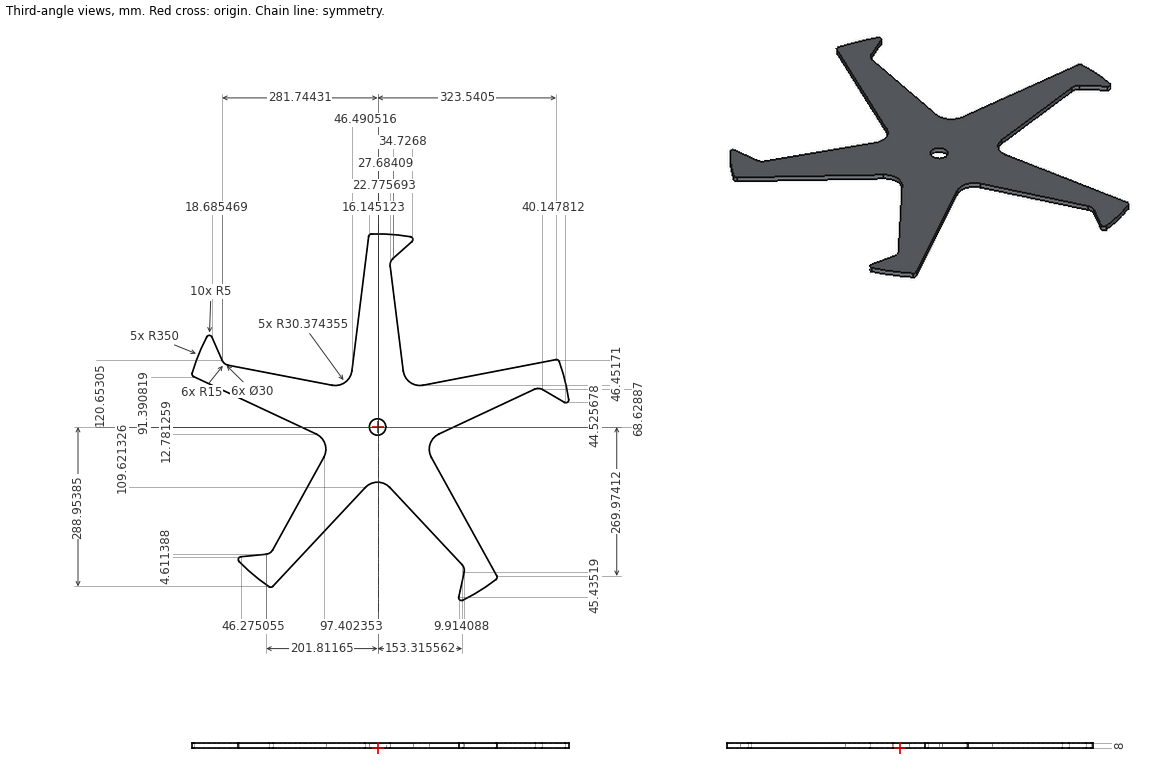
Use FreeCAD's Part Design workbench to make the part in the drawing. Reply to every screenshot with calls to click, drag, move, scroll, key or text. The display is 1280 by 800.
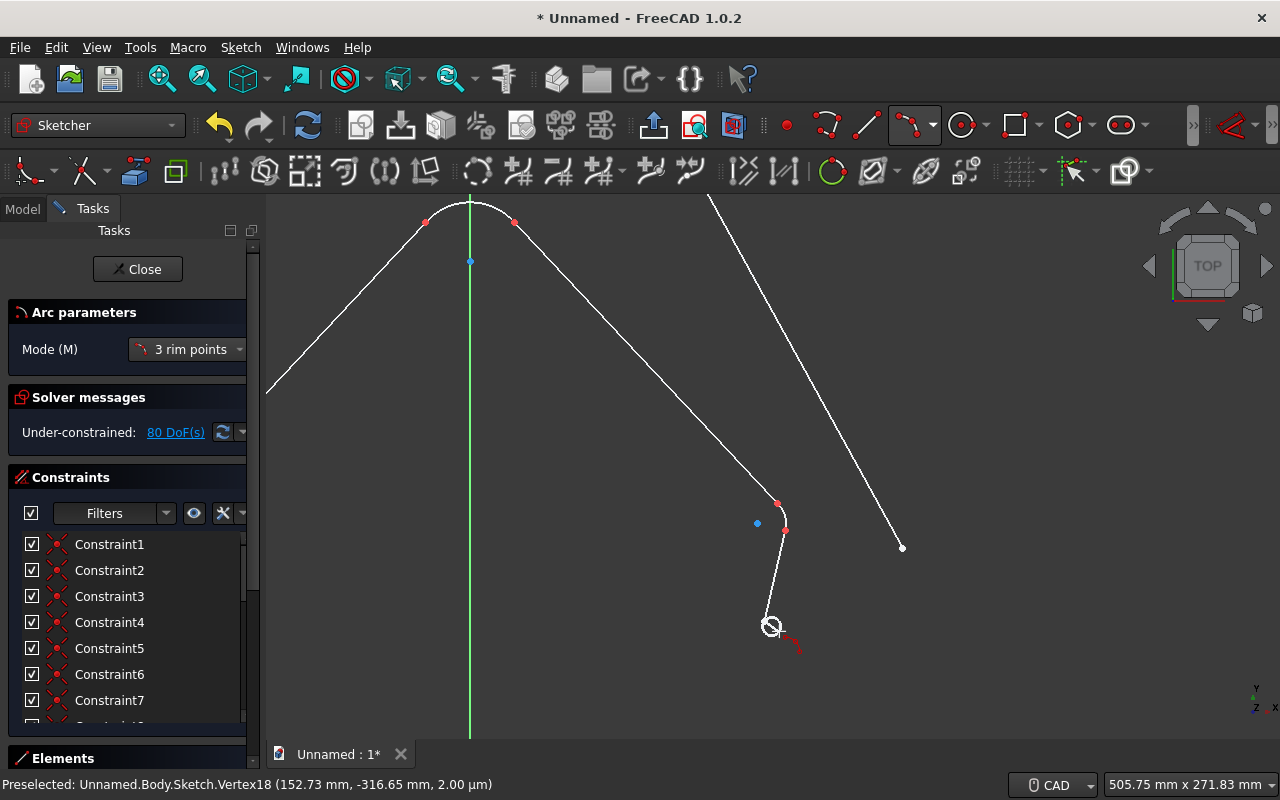
scroll(769, 630, up, 6)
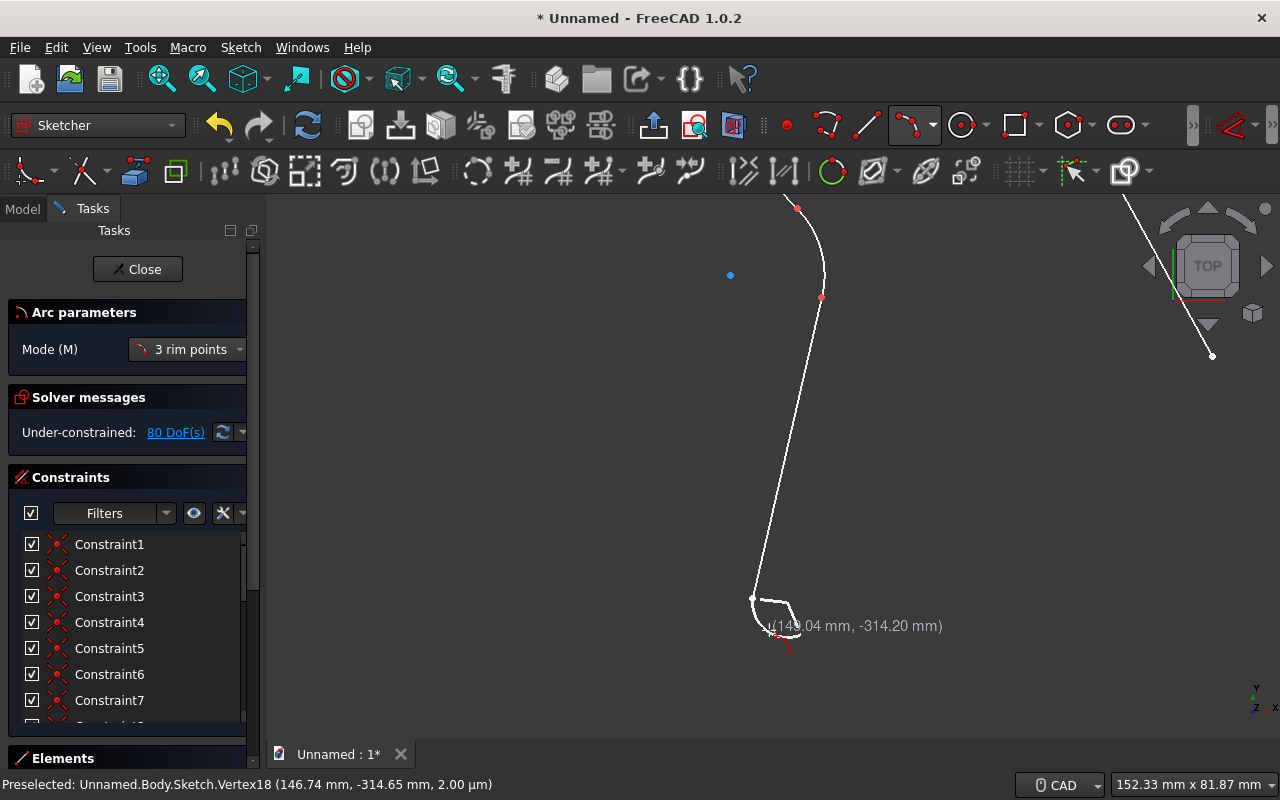
click(767, 628)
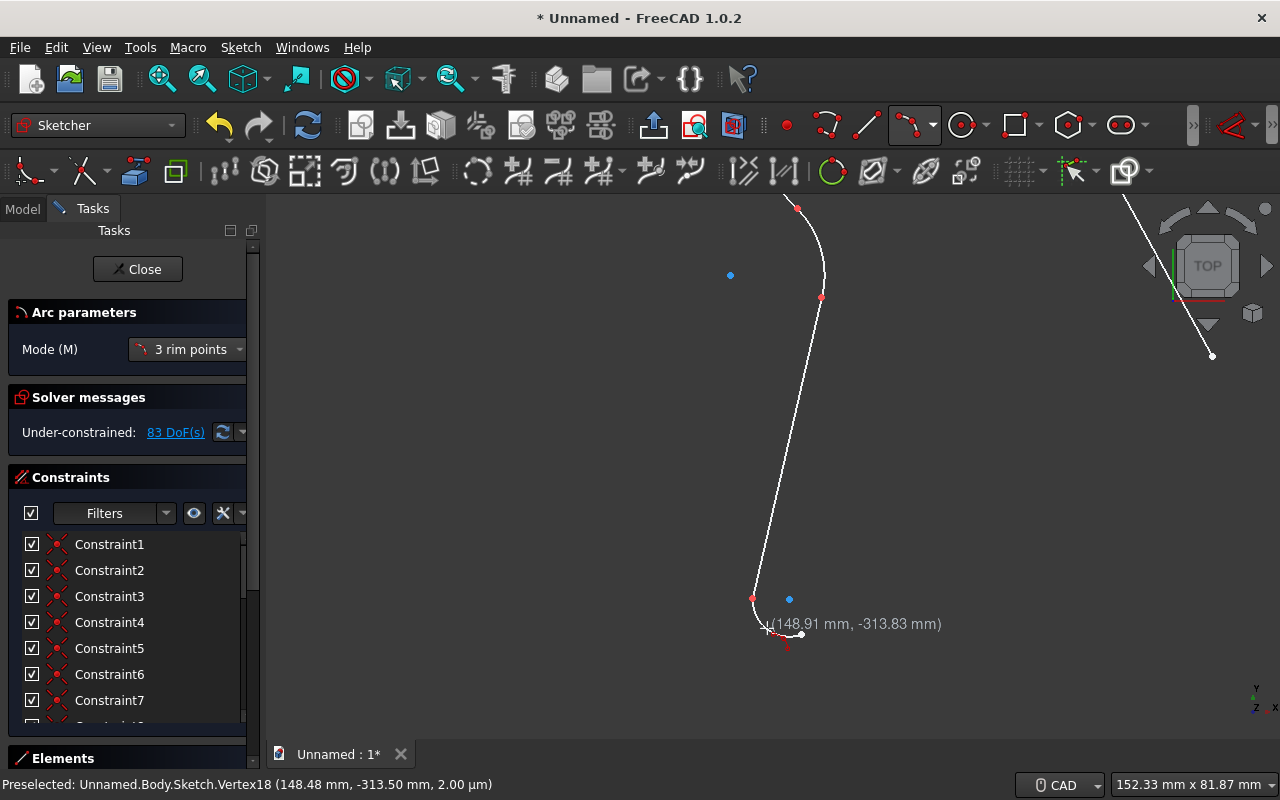
click(801, 635)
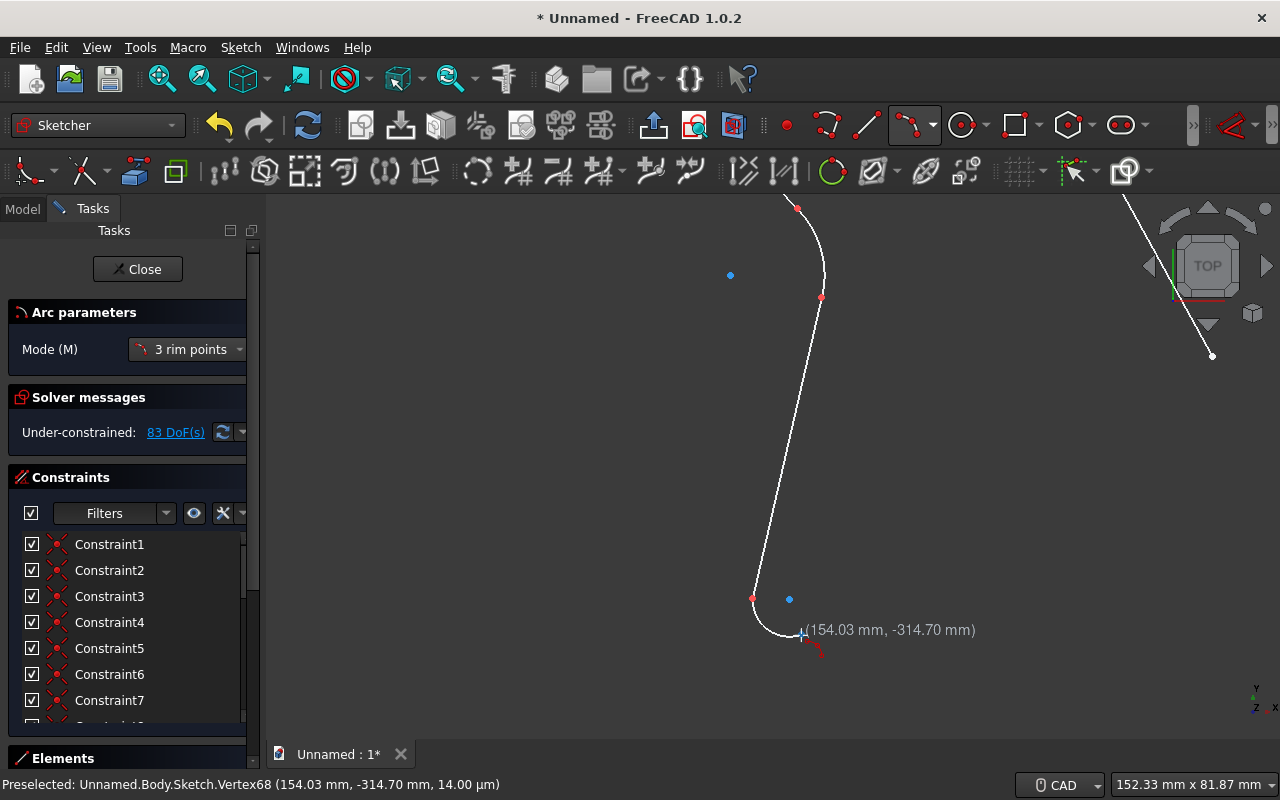
scroll(776, 631, down, 13)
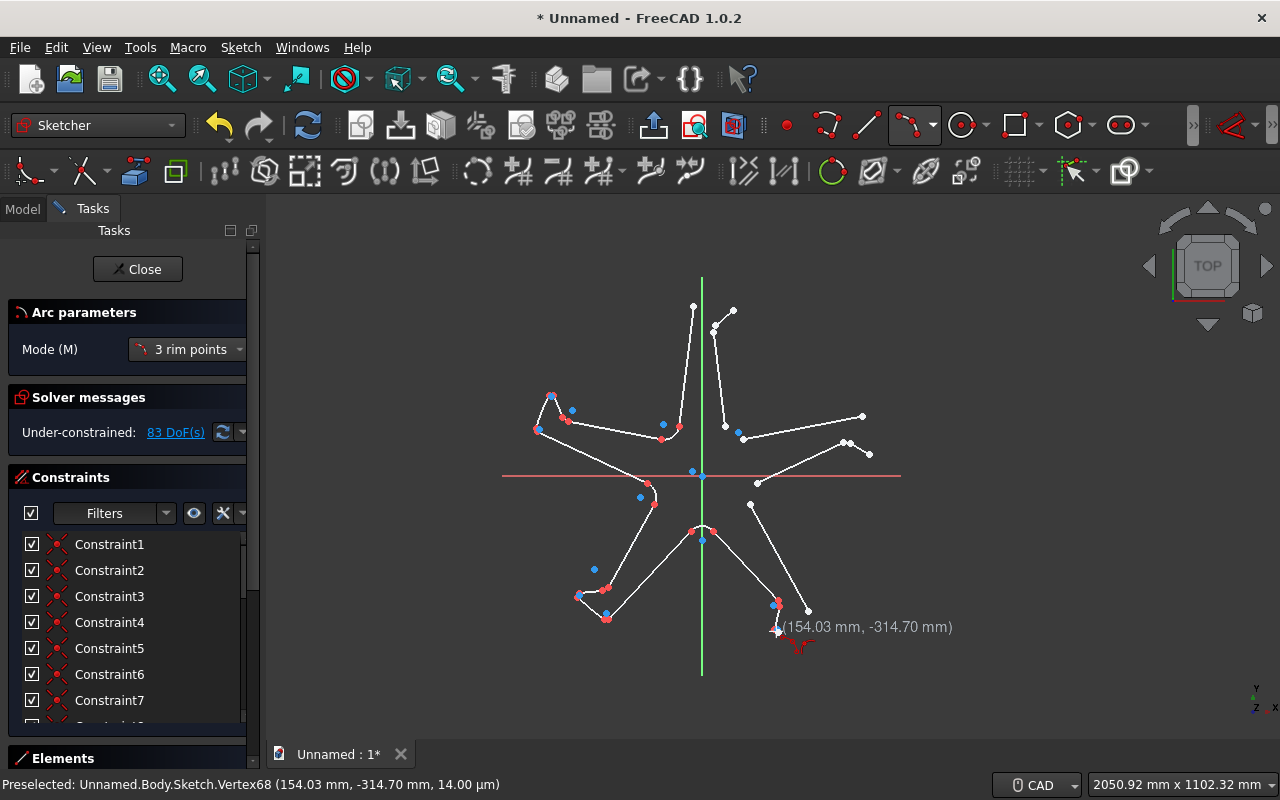
scroll(808, 613, up, 8)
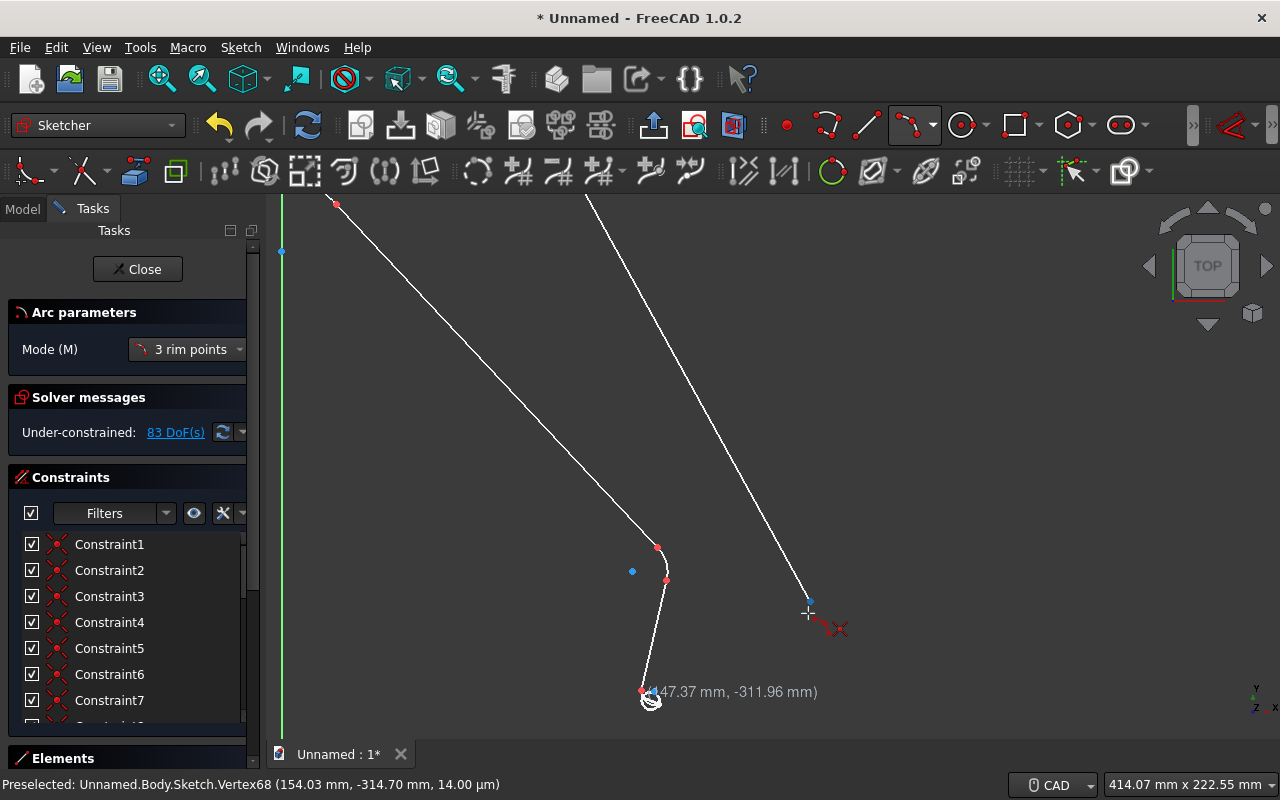
click(808, 610)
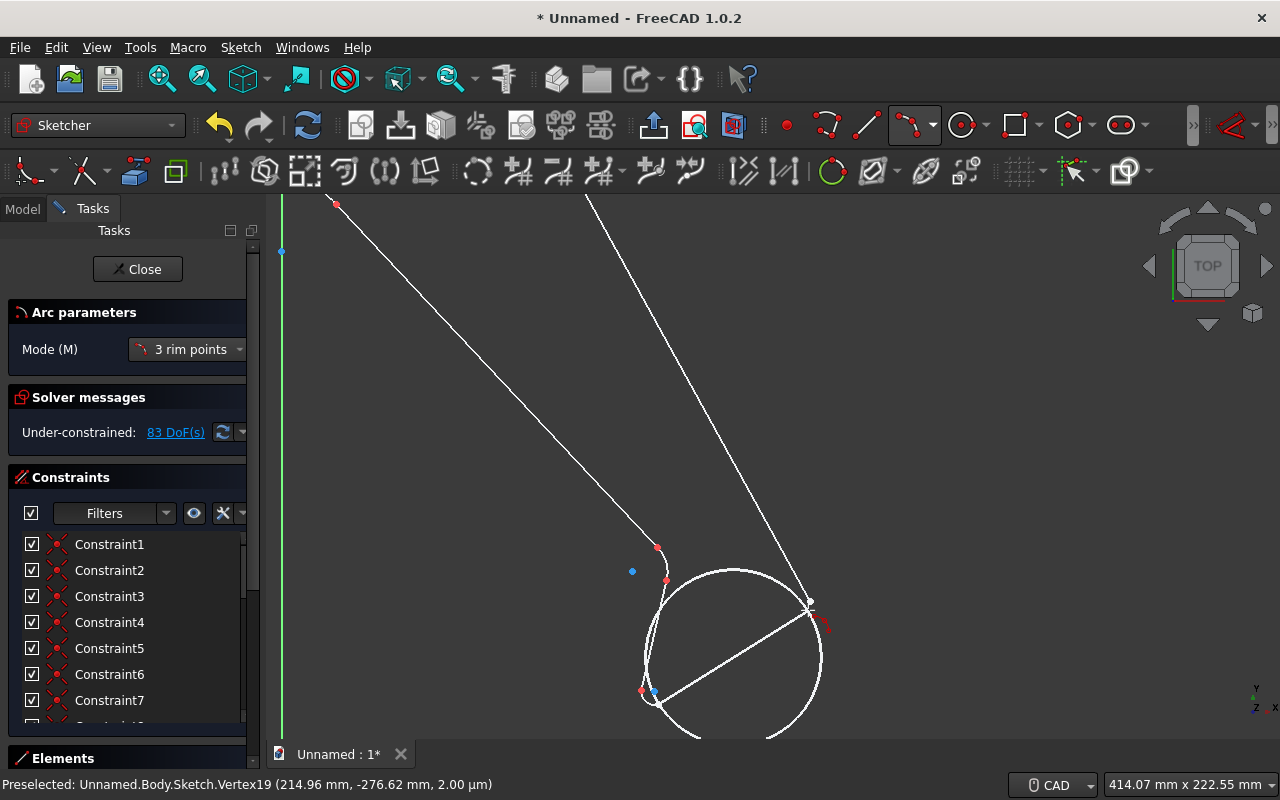
scroll(736, 660, up, 7)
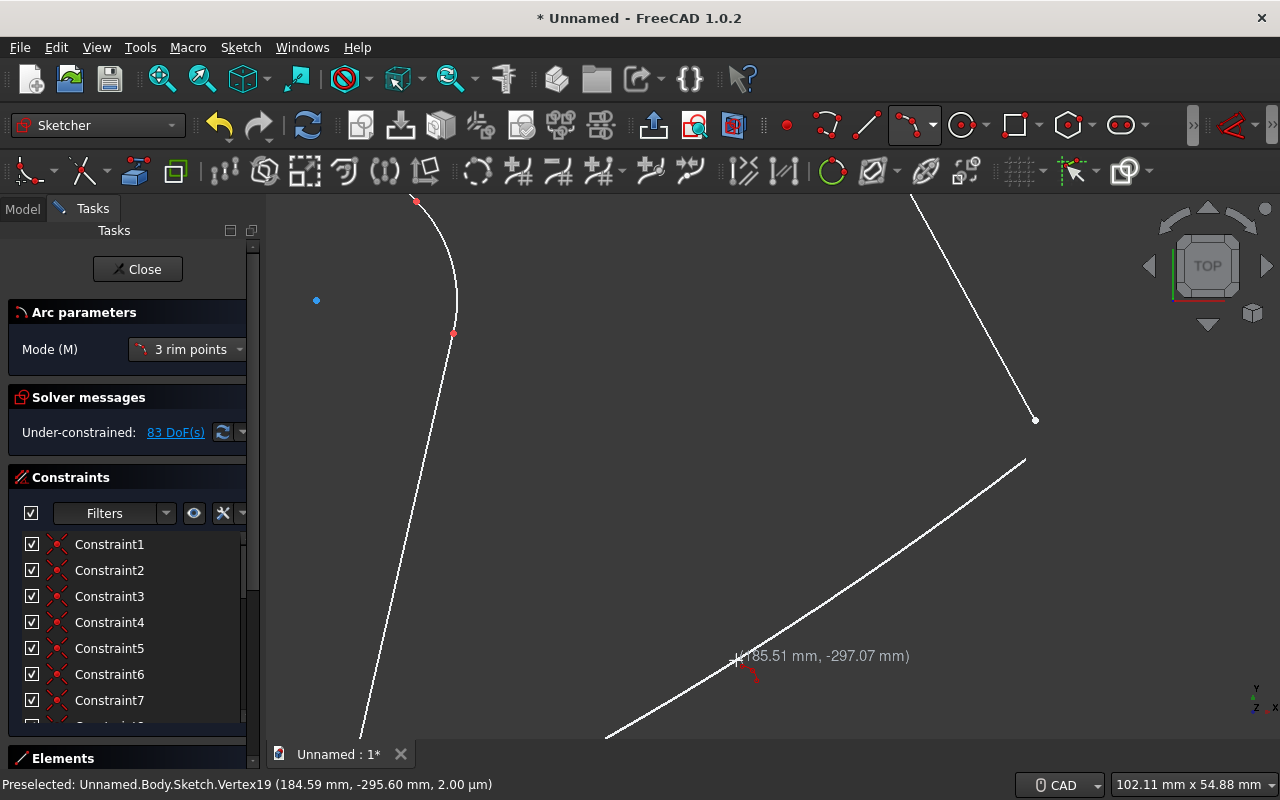
click(734, 659)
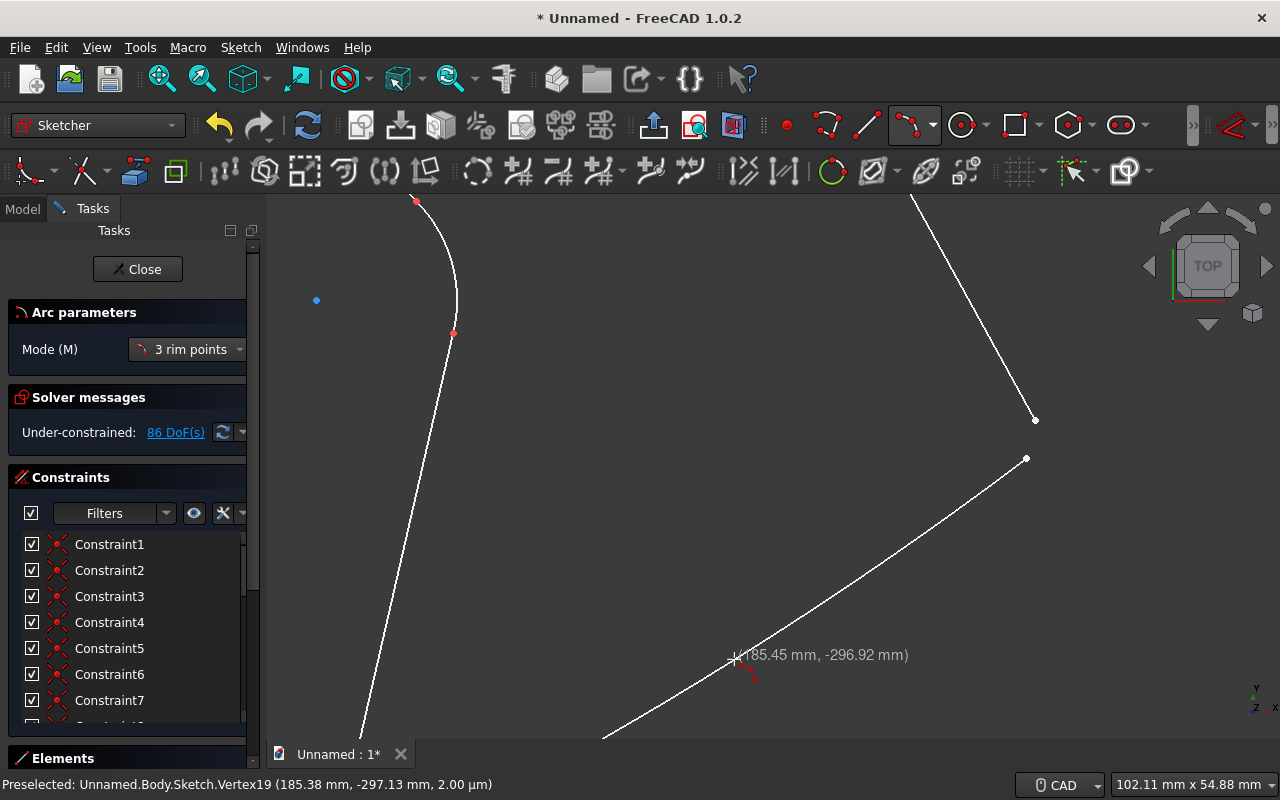
scroll(797, 620, down, 15)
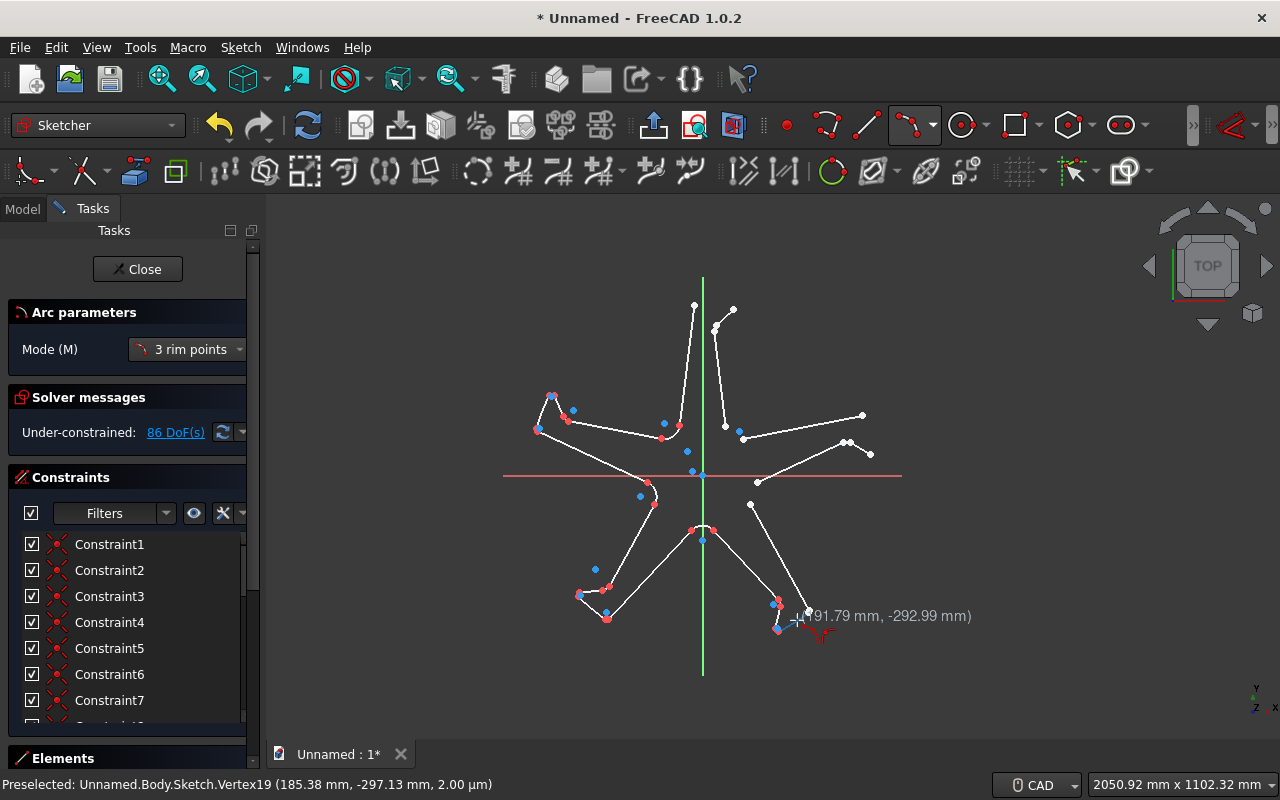
scroll(809, 613, up, 8)